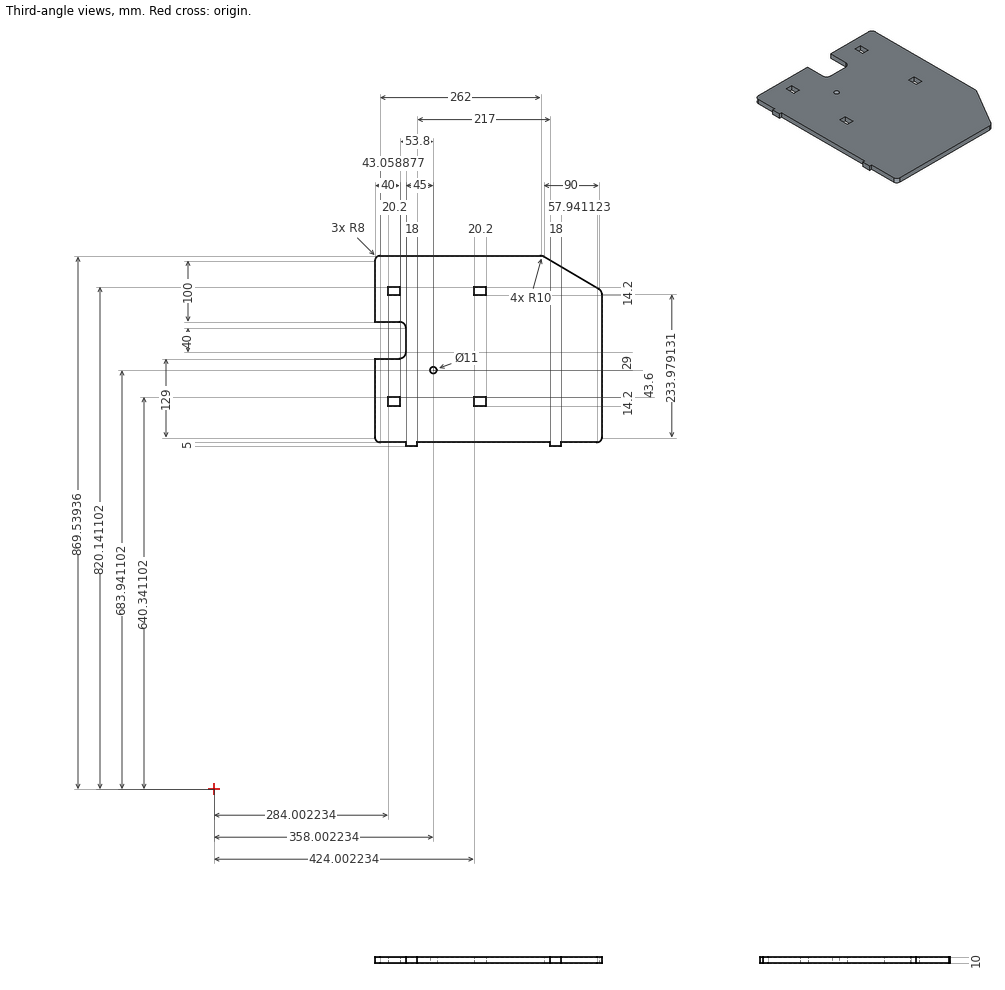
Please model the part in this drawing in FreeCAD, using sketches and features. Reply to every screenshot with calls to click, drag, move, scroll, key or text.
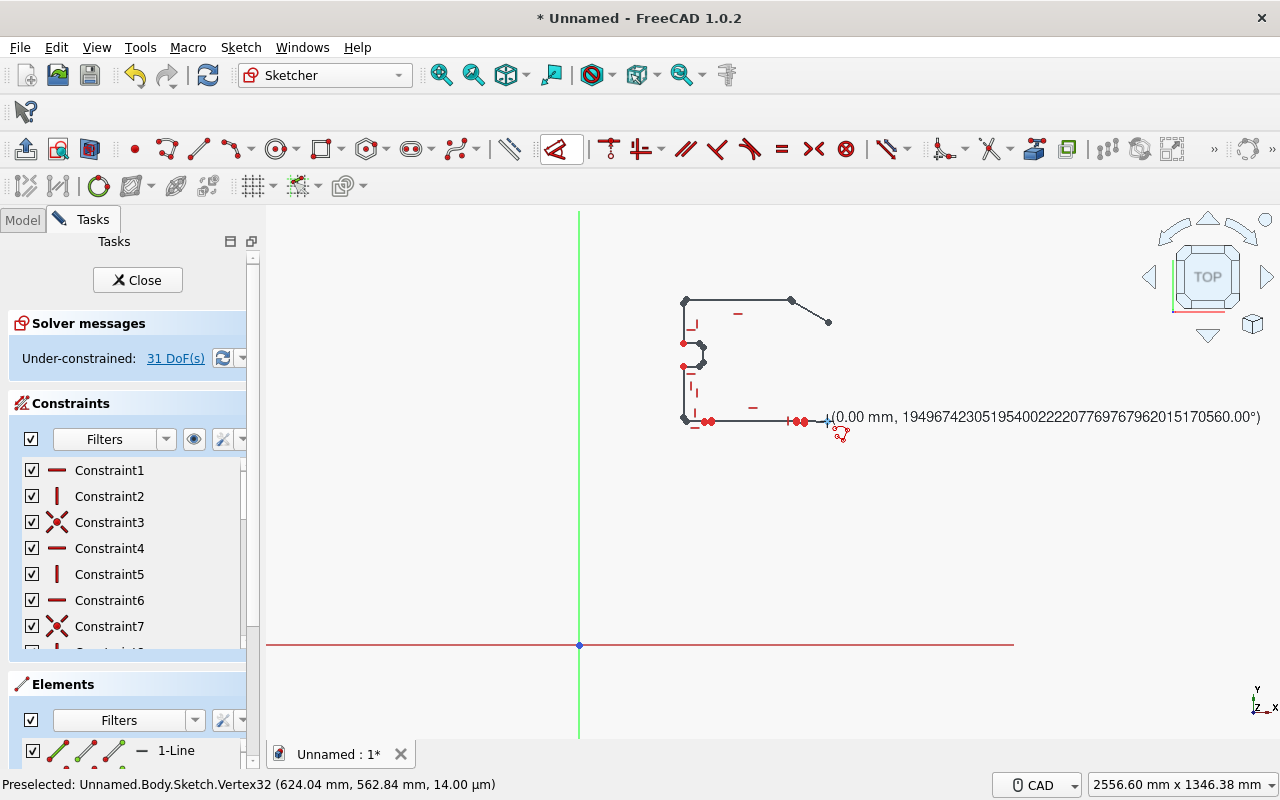
click(200, 150)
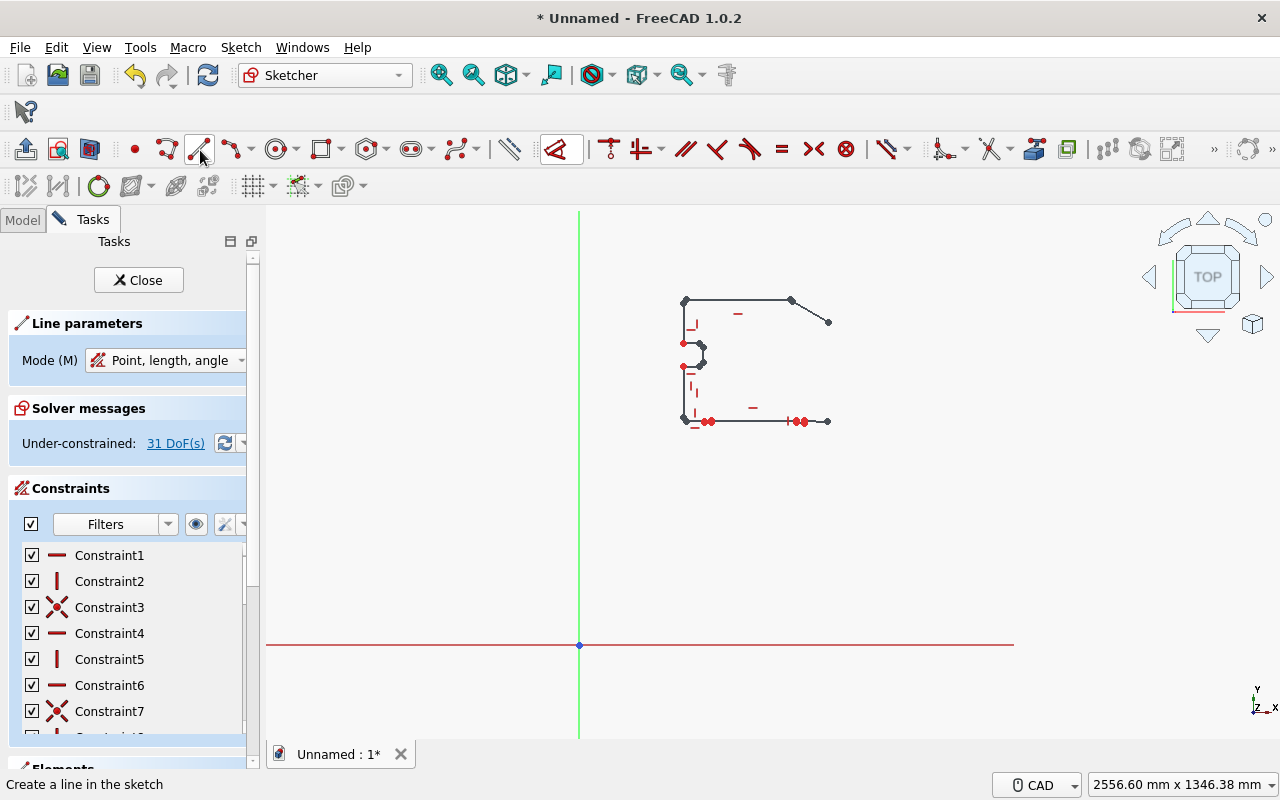
scroll(831, 418, up, 7)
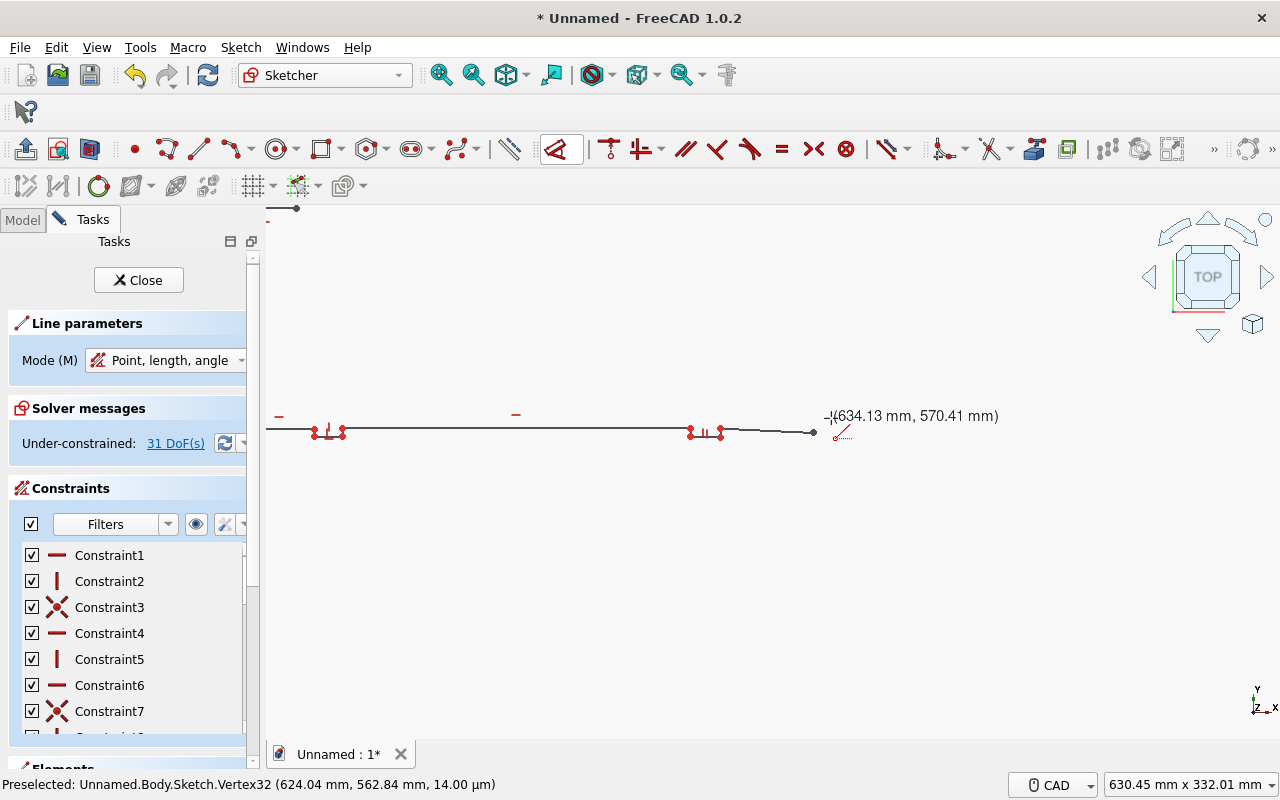
click(827, 415)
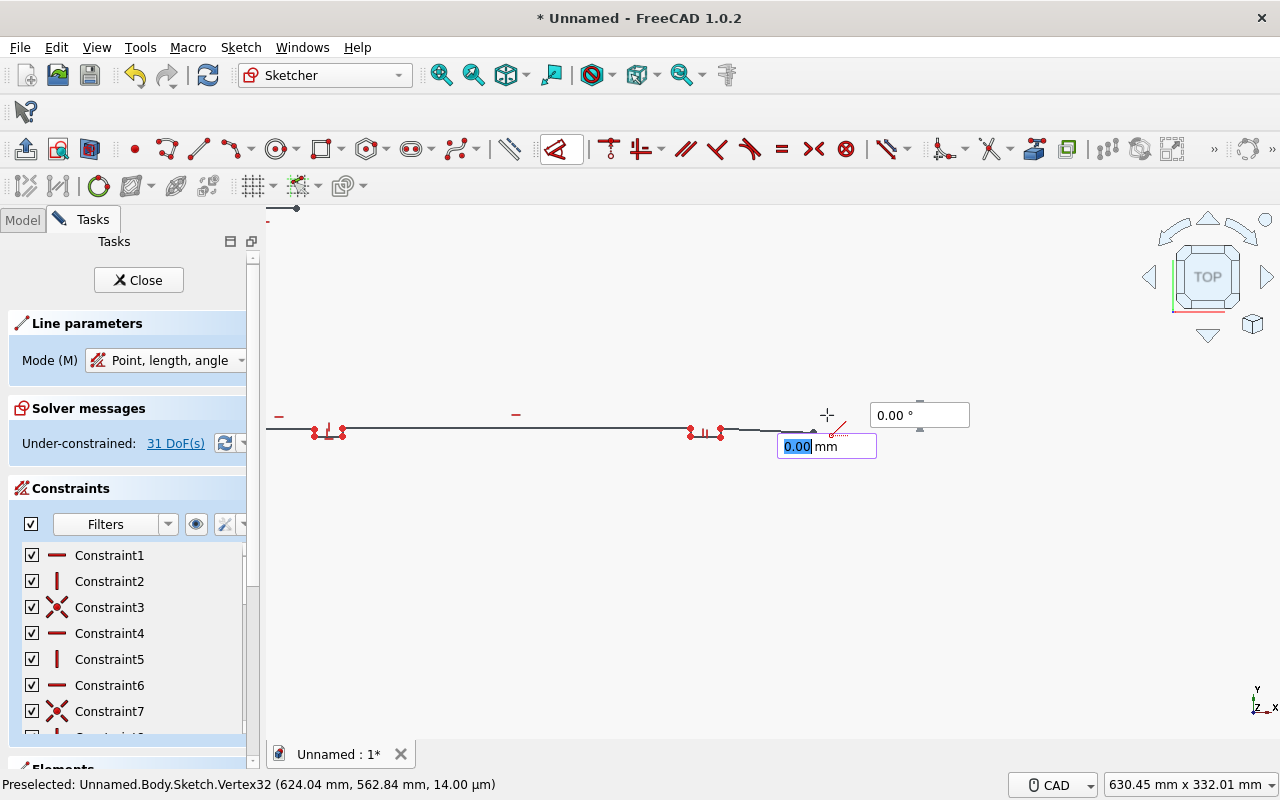
scroll(831, 418, down, 7)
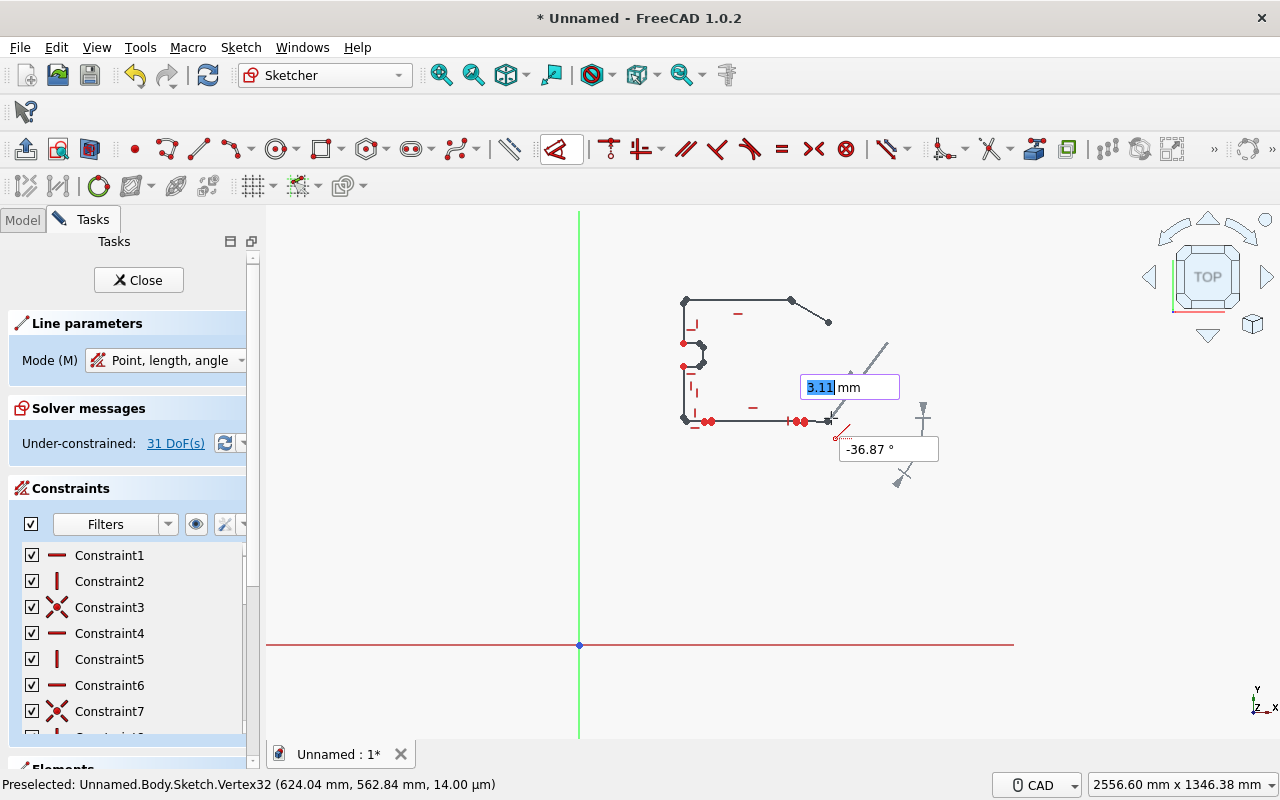
scroll(831, 325, up, 7)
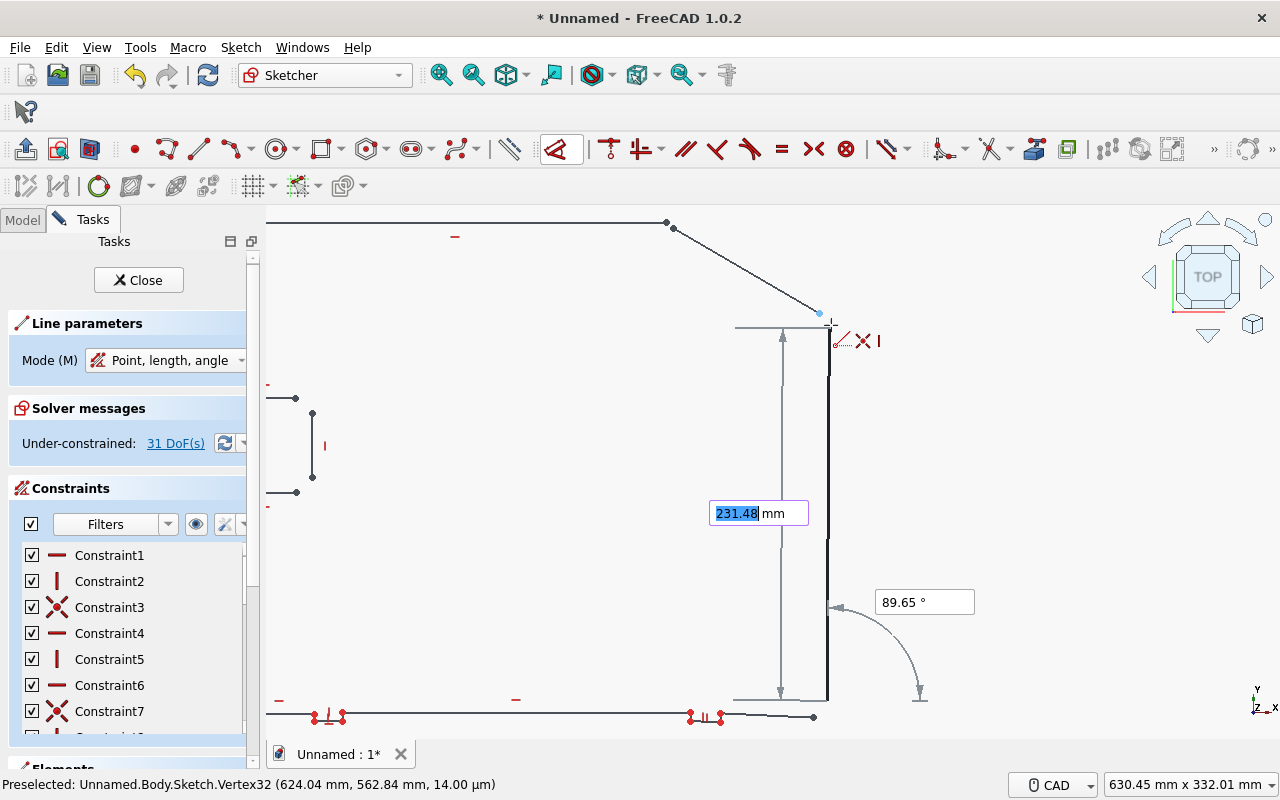
click(827, 323)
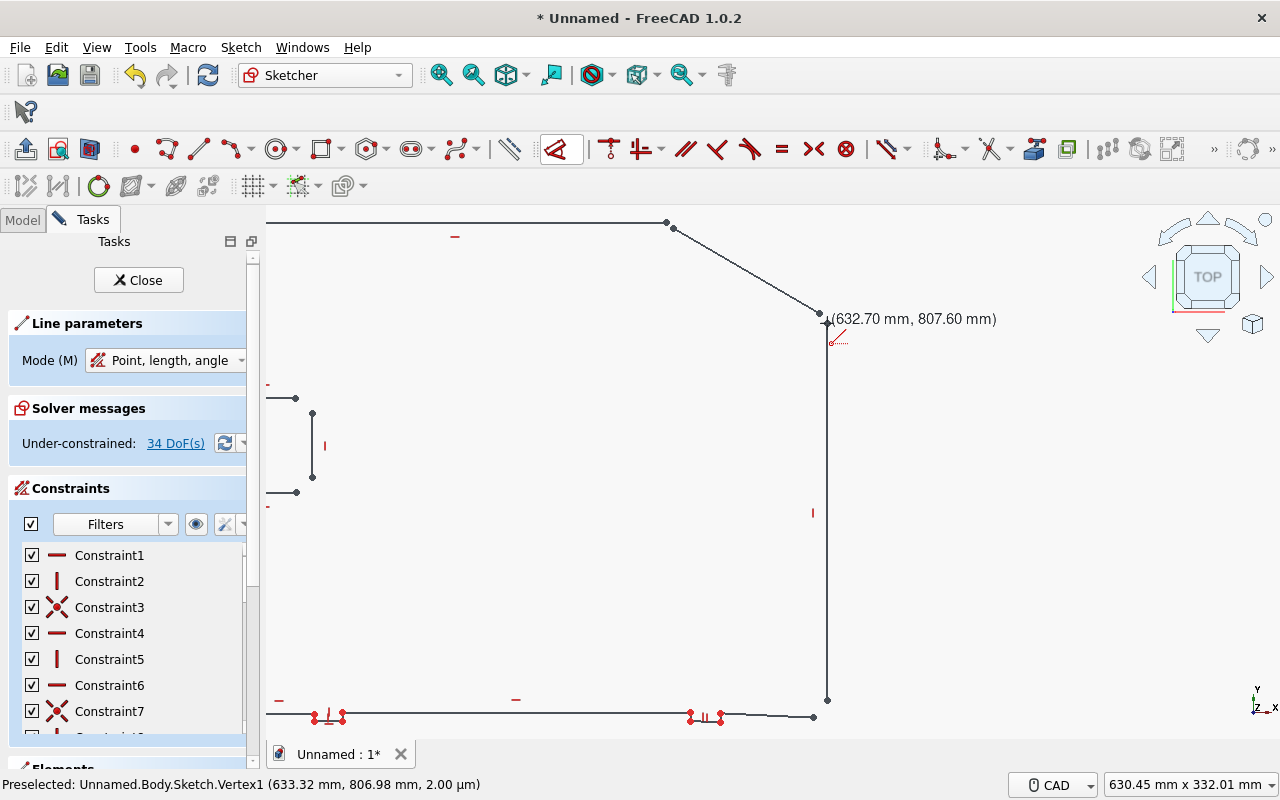
click(232, 150)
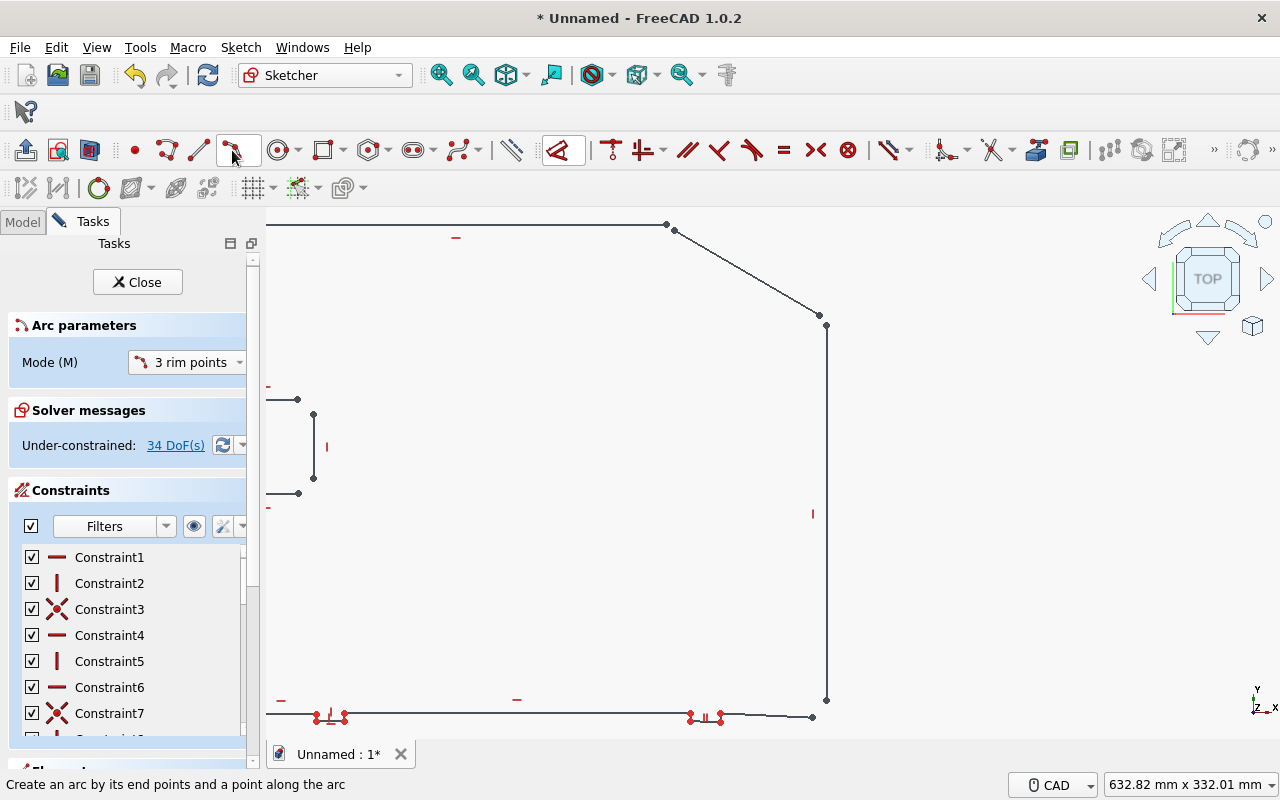
scroll(830, 326, down, 7)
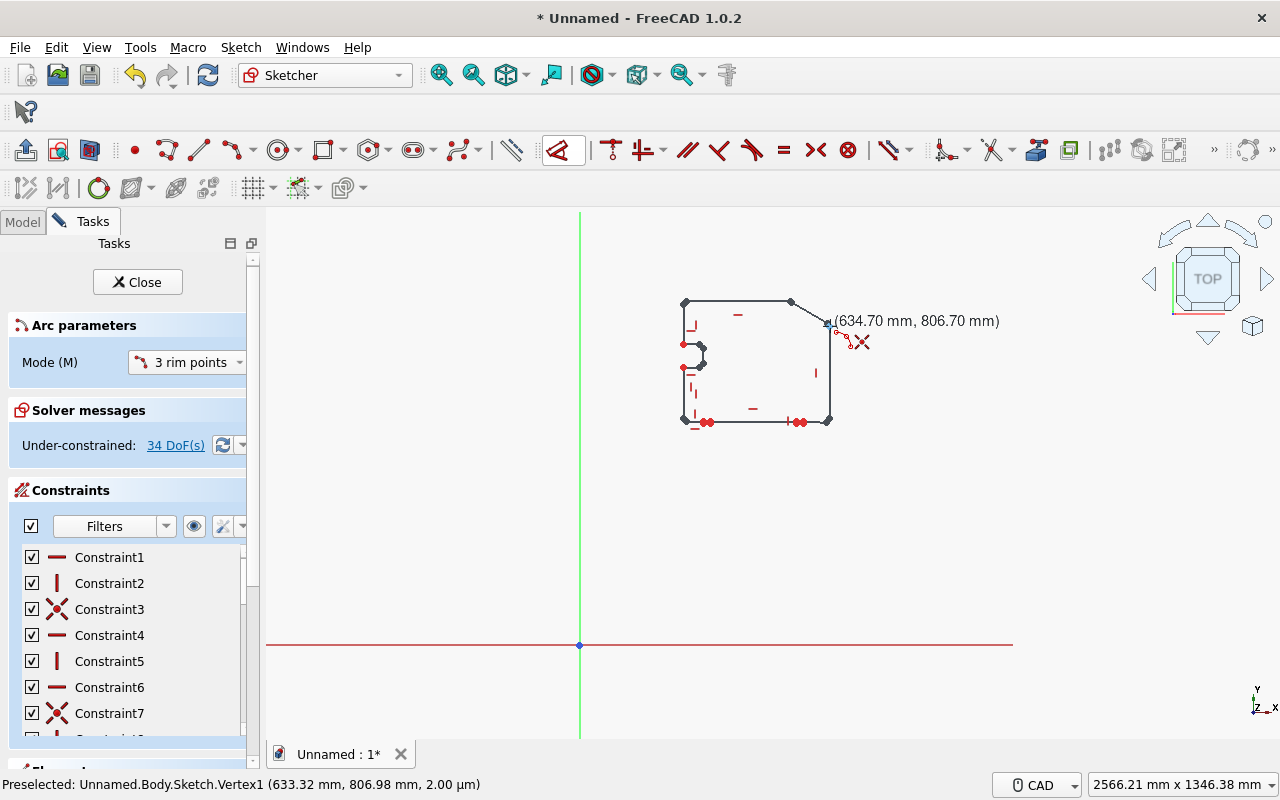
scroll(792, 302, up, 11)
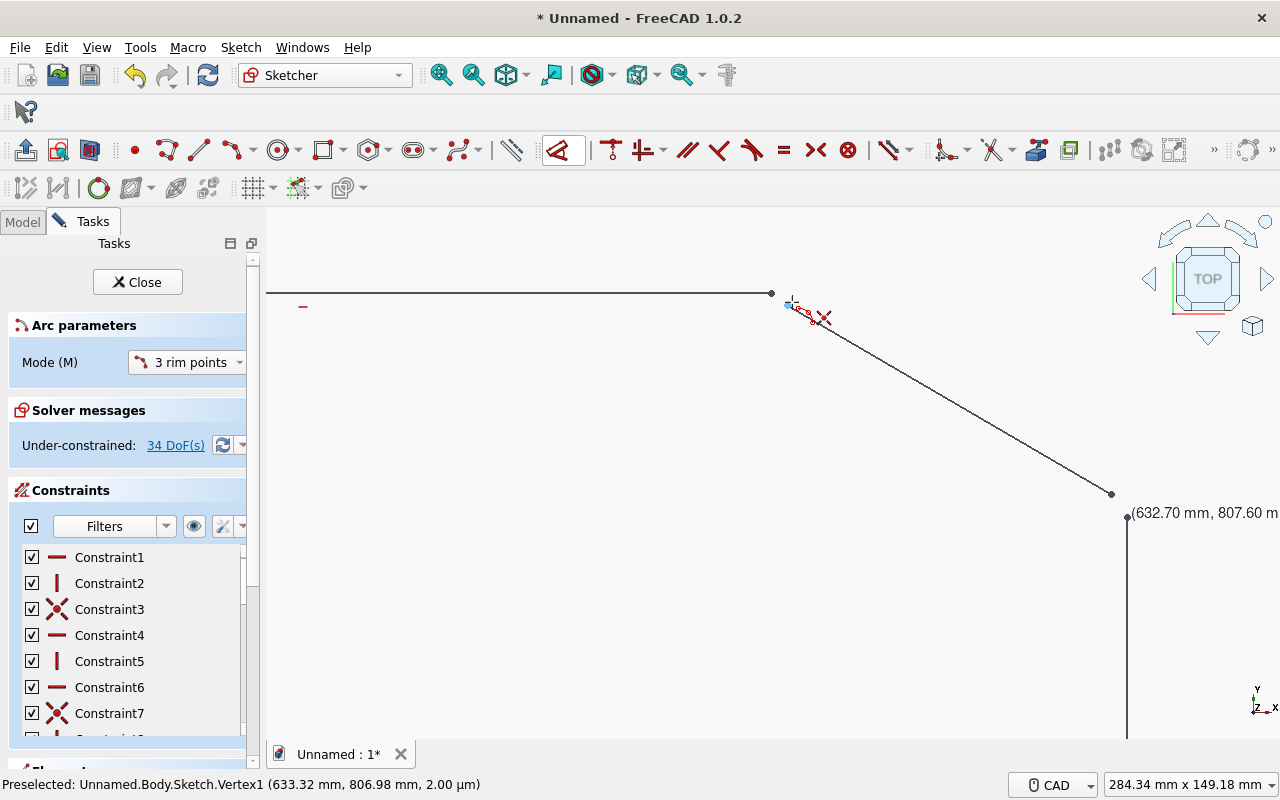
click(787, 306)
click(772, 293)